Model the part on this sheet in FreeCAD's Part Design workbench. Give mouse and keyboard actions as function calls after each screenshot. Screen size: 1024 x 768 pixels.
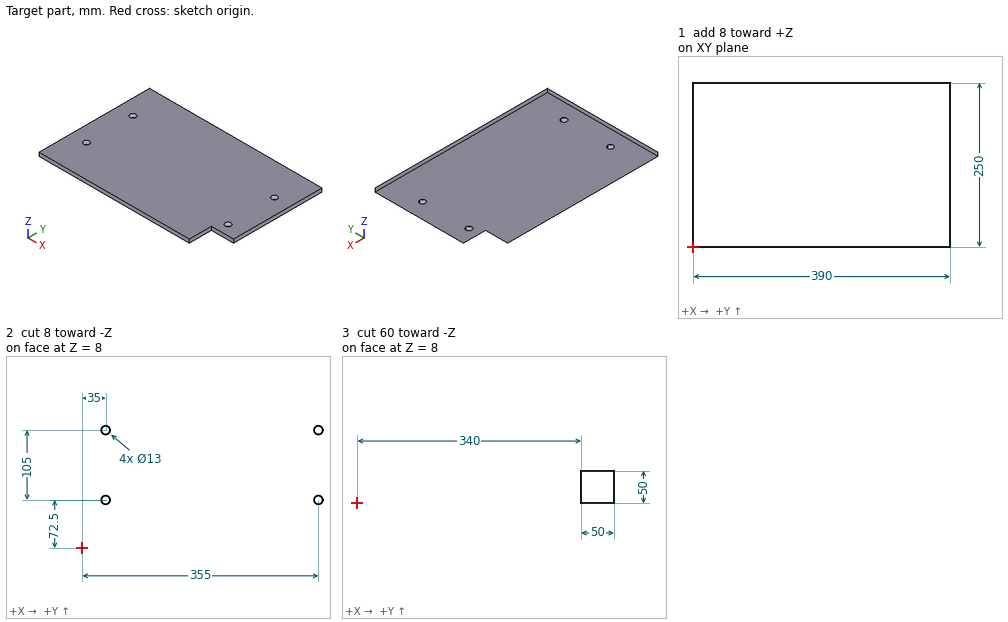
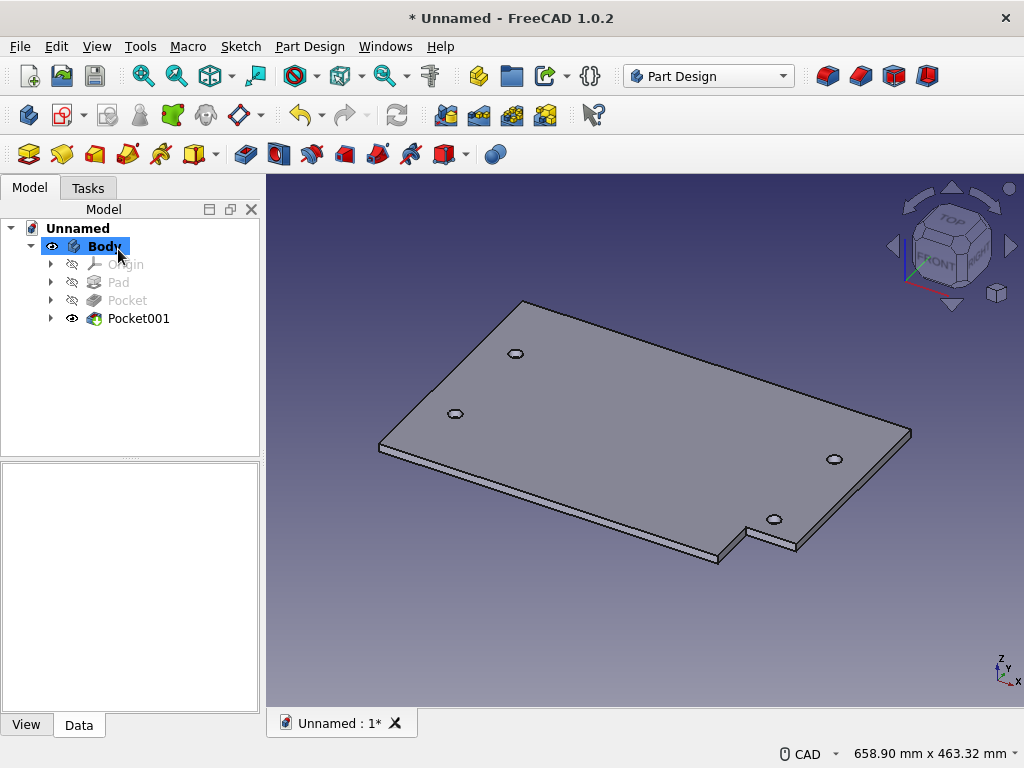
key(0)